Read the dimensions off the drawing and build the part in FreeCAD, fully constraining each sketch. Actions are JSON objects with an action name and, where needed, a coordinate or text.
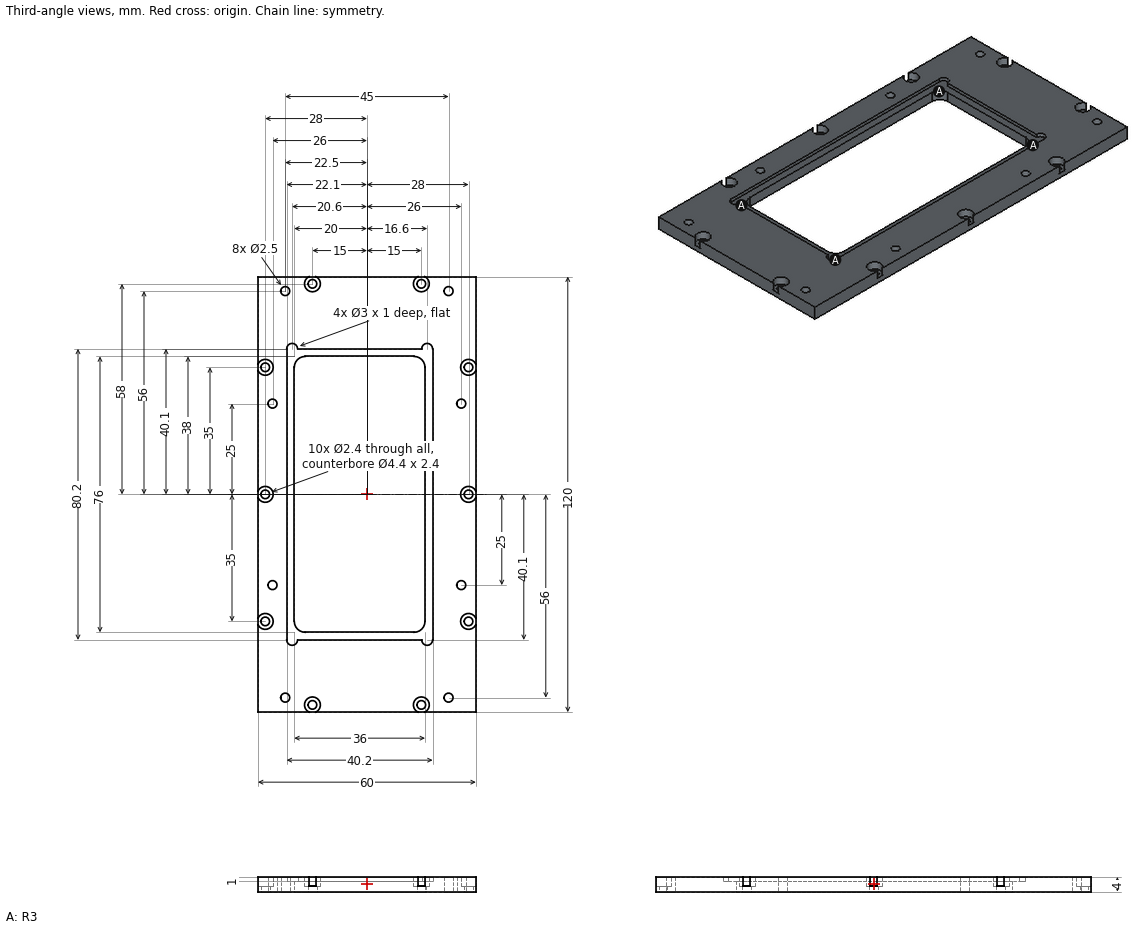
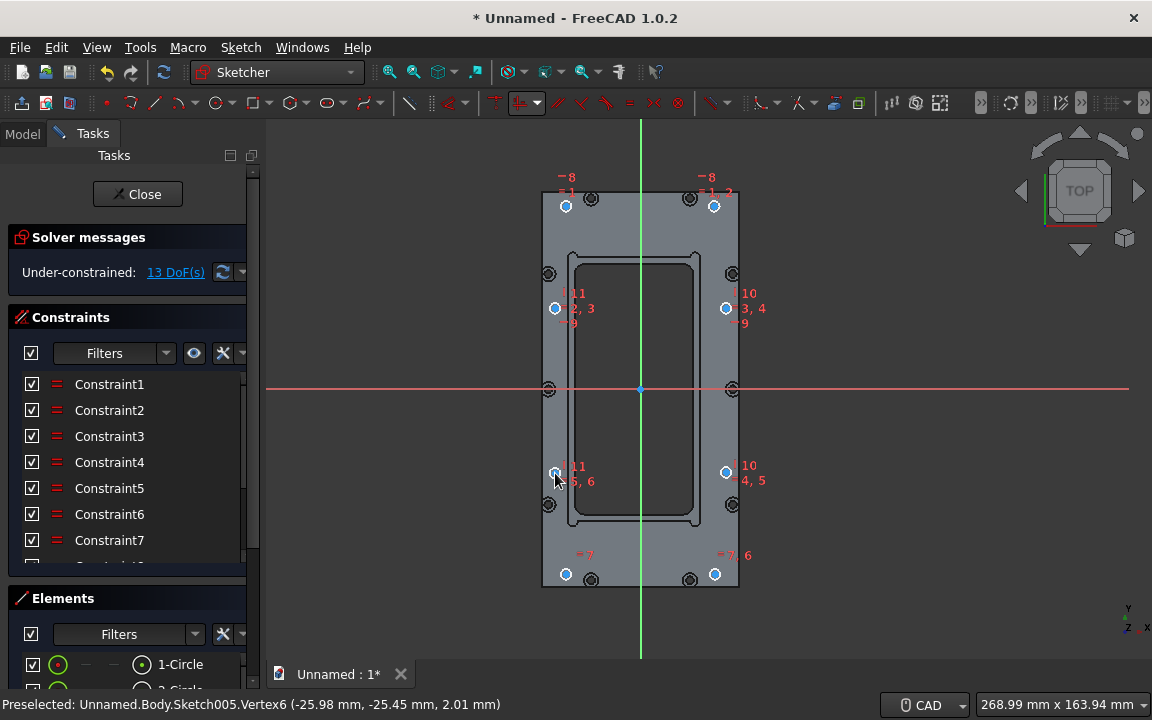
{"action": "left_click", "coordinate": [726, 472]}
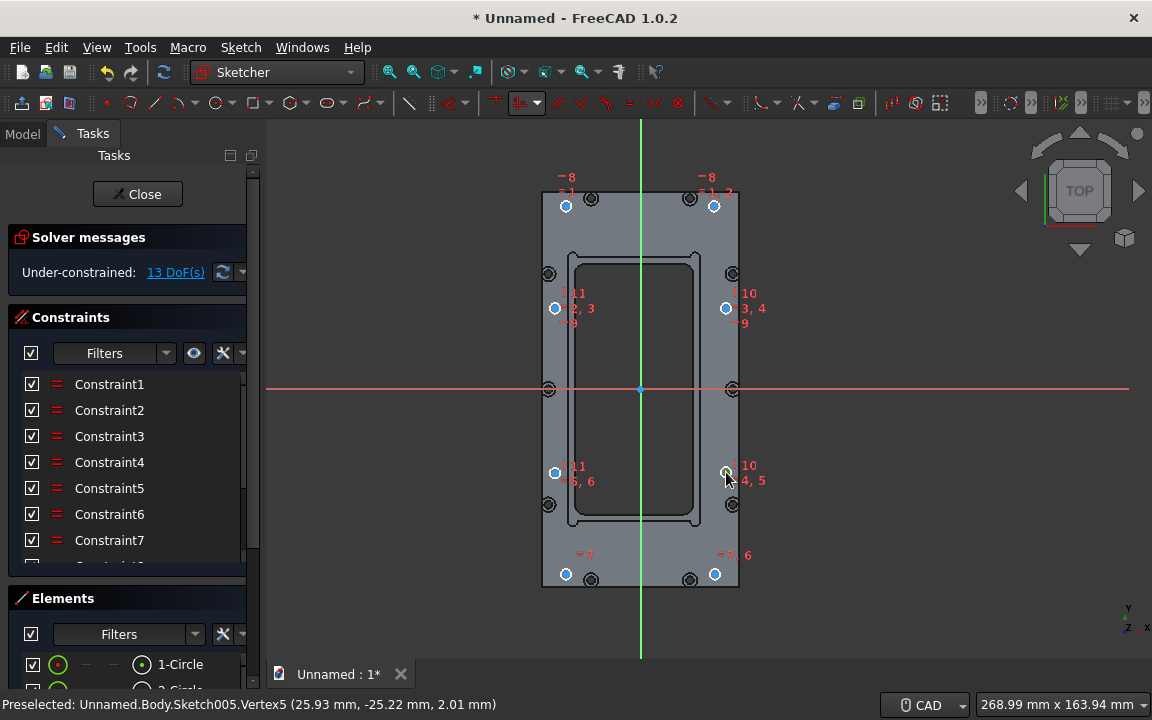
{"action": "left_click", "coordinate": [555, 473]}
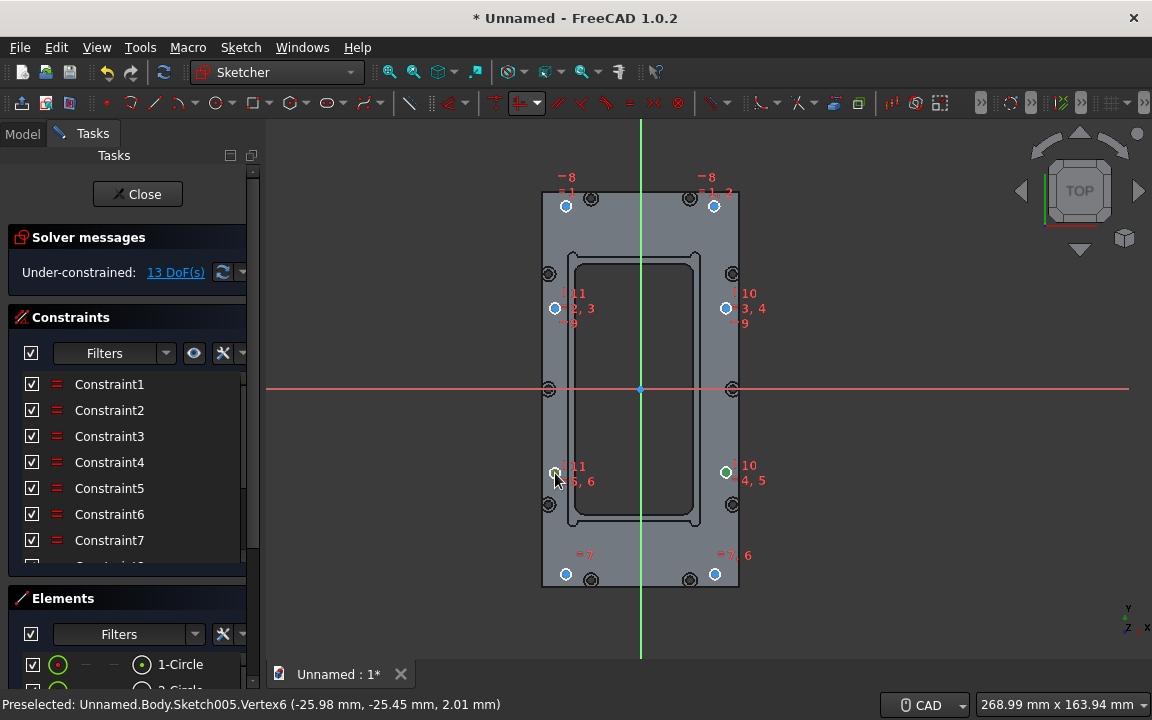
{"action": "key", "text": "h"}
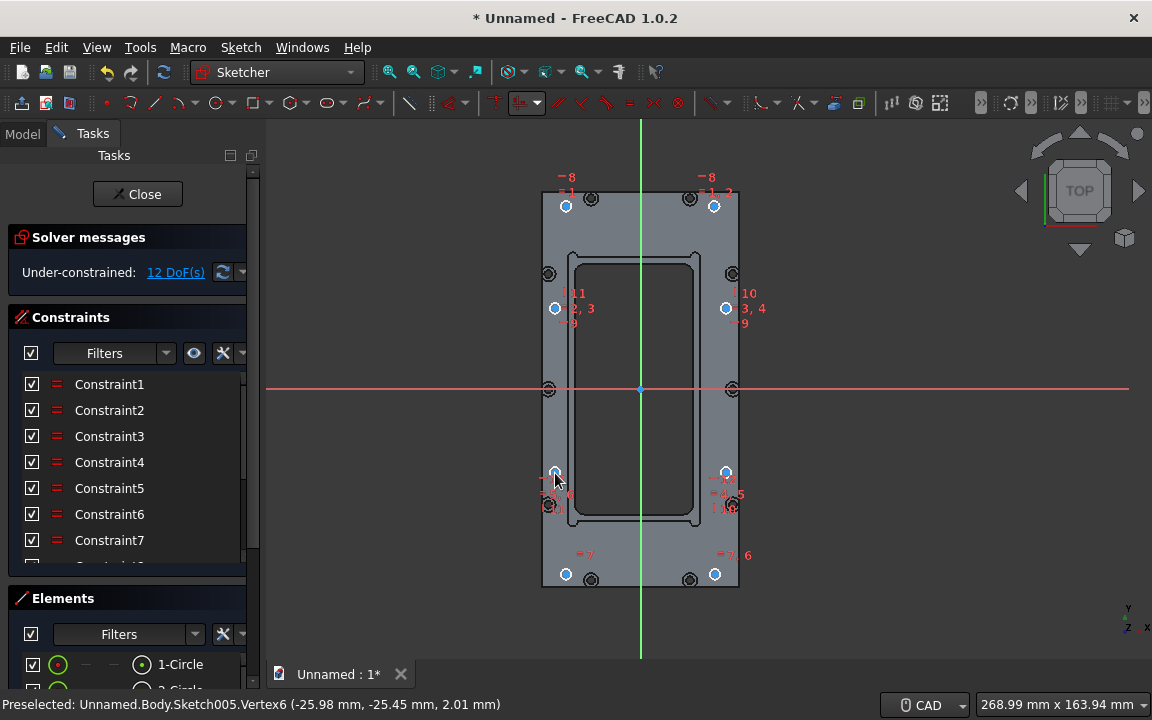
{"action": "left_click", "coordinate": [714, 206]}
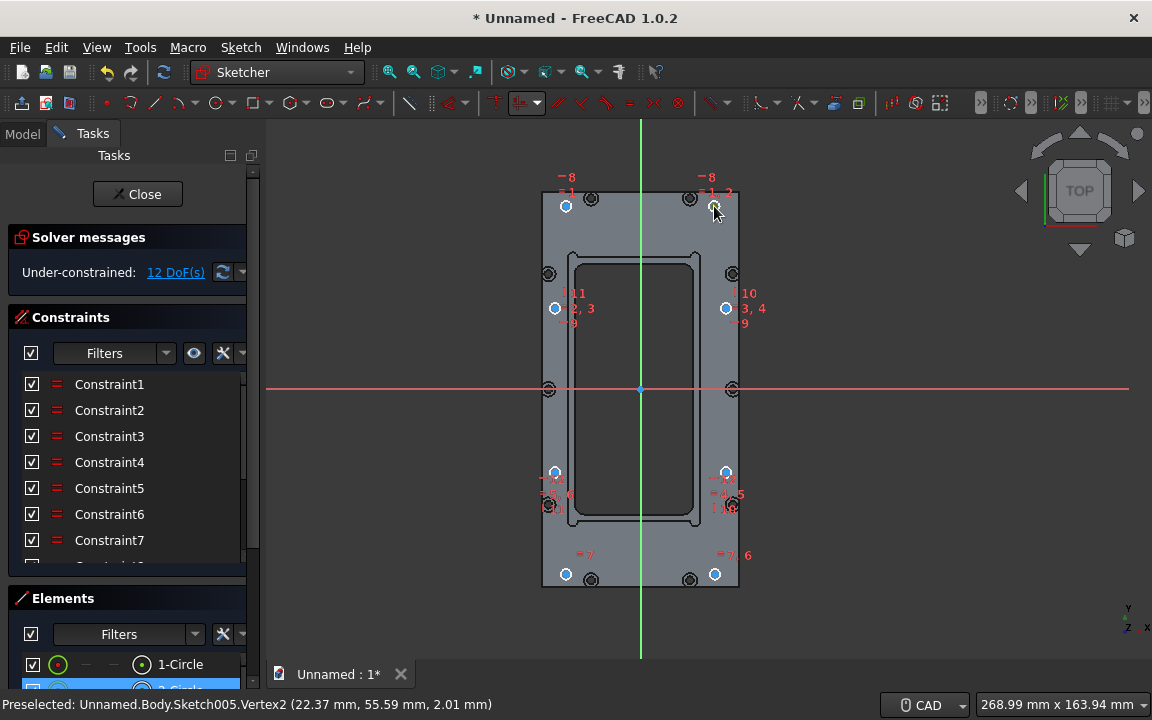
{"action": "left_click", "coordinate": [715, 574]}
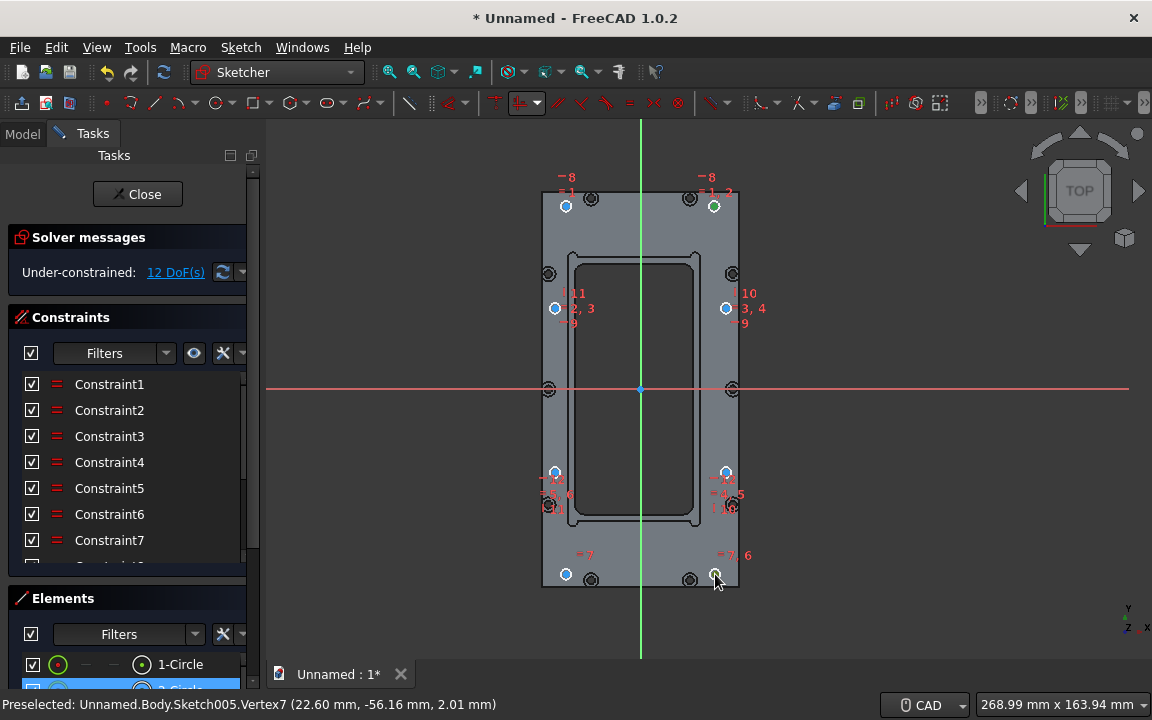
{"action": "key", "text": "v"}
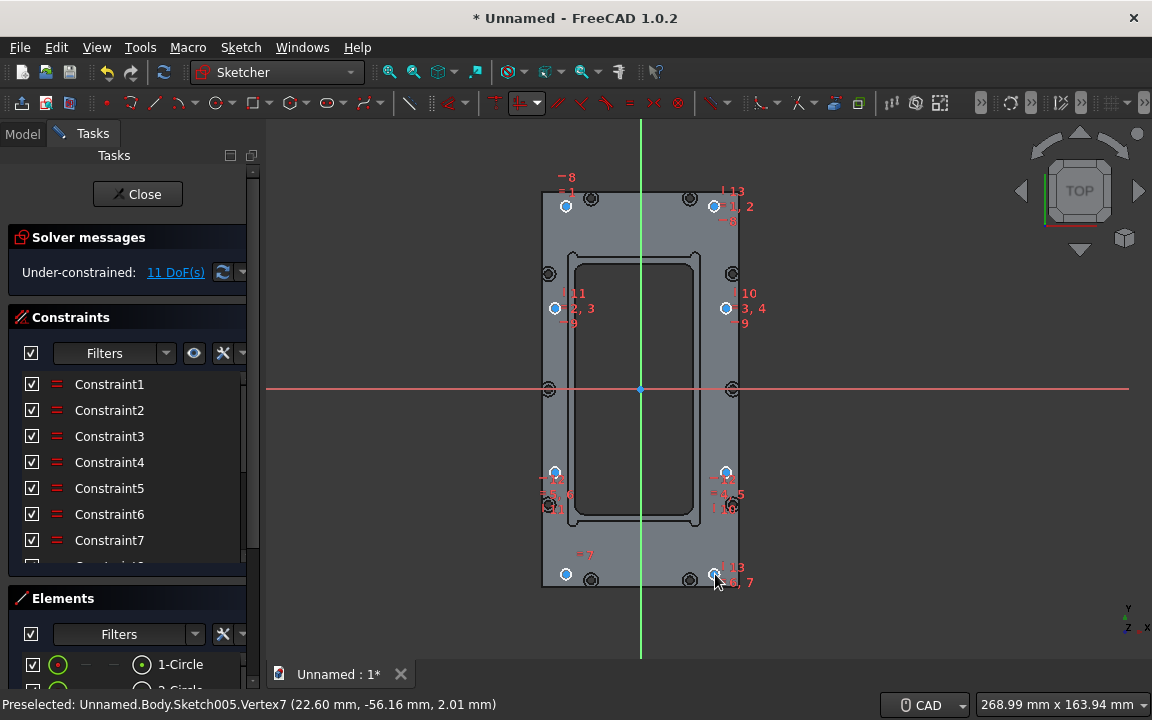
{"action": "left_click", "coordinate": [566, 206]}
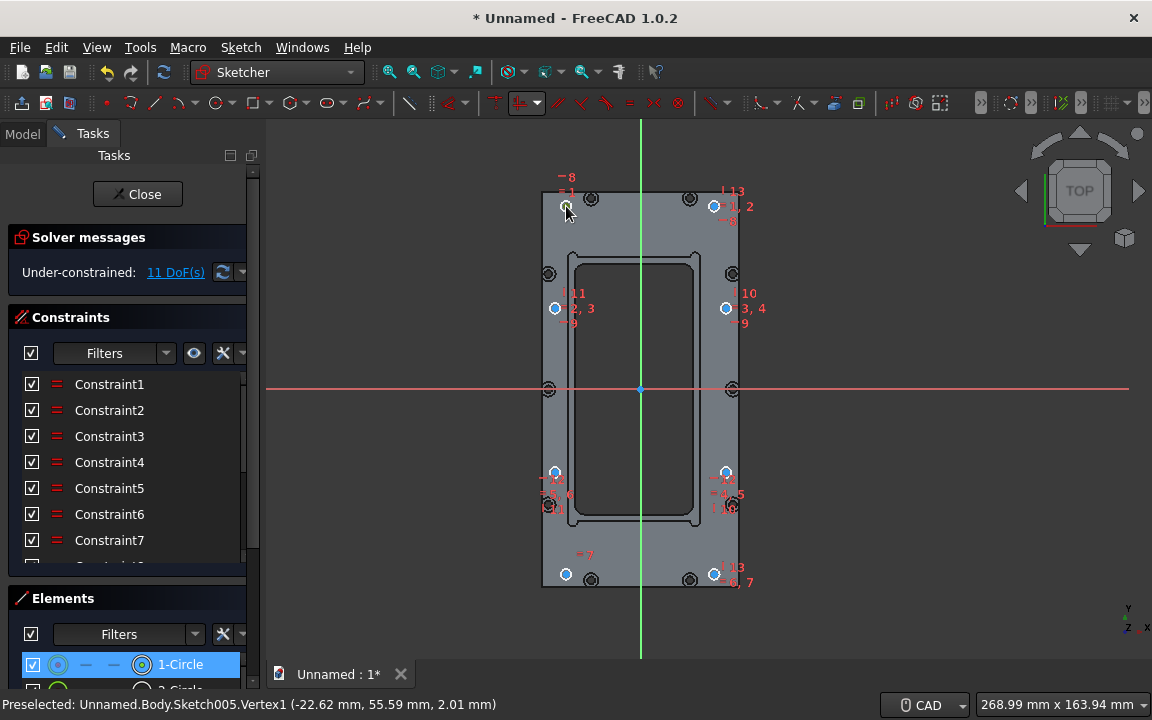
{"action": "left_click", "coordinate": [566, 574]}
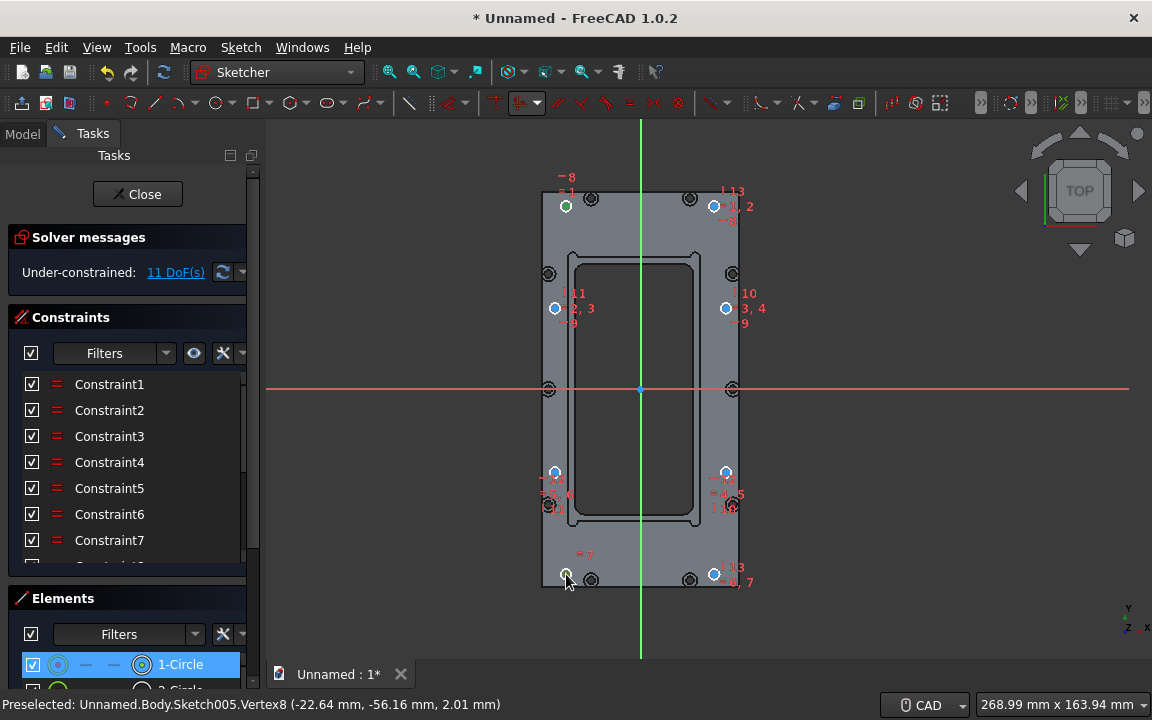
{"action": "key", "text": "v"}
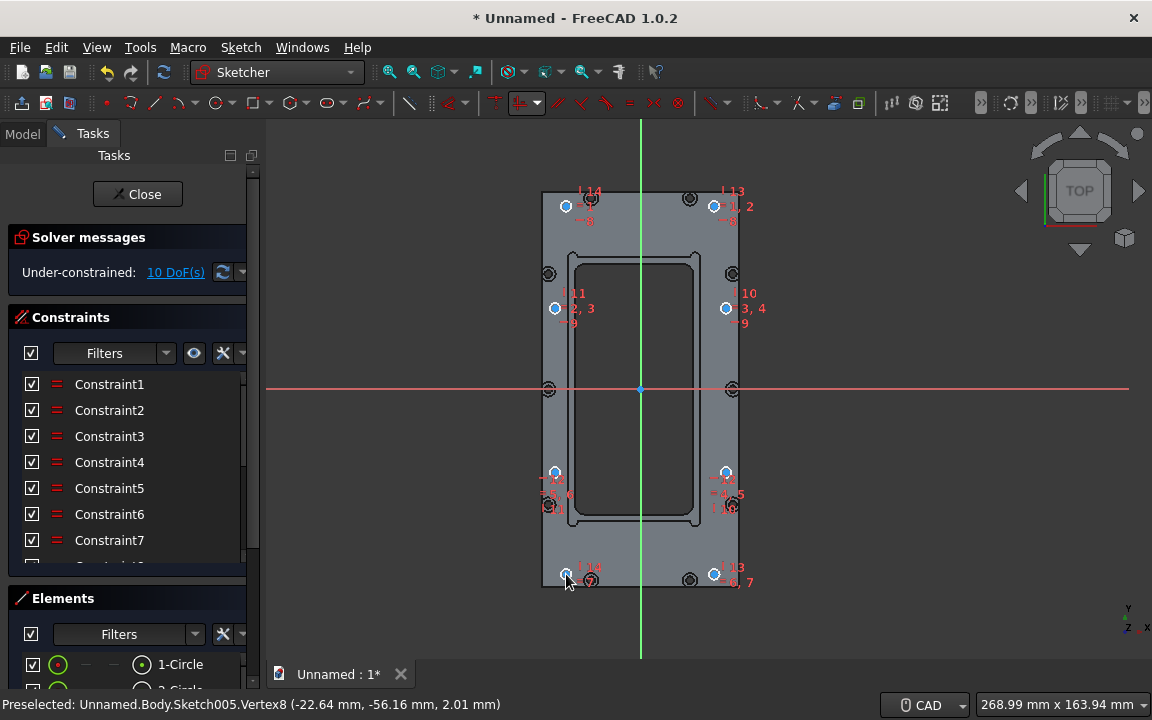
{"action": "left_click", "coordinate": [714, 574]}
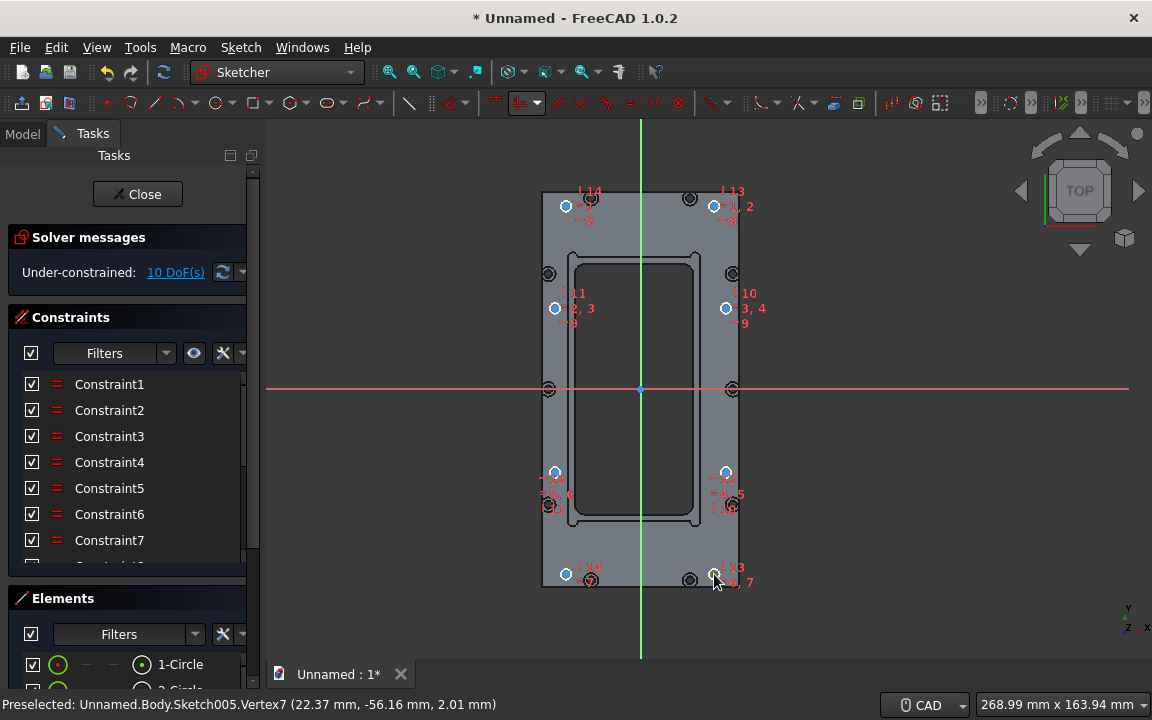
{"action": "left_click", "coordinate": [566, 574]}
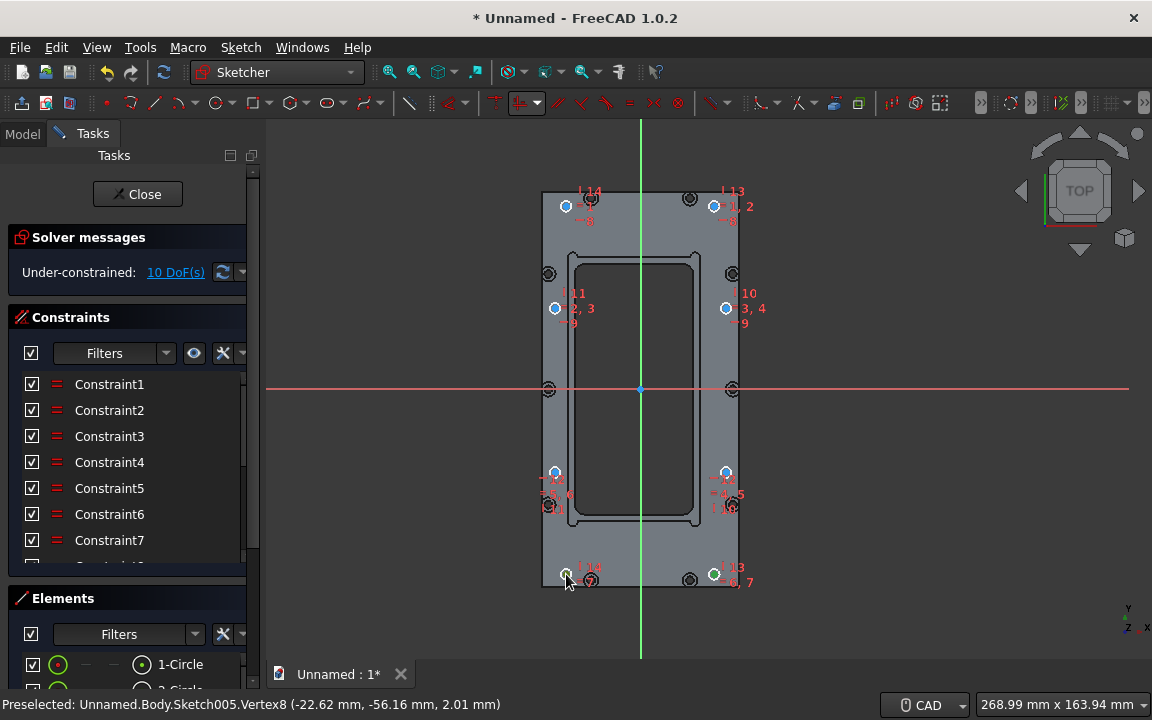
{"action": "left_click", "coordinate": [540, 104]}